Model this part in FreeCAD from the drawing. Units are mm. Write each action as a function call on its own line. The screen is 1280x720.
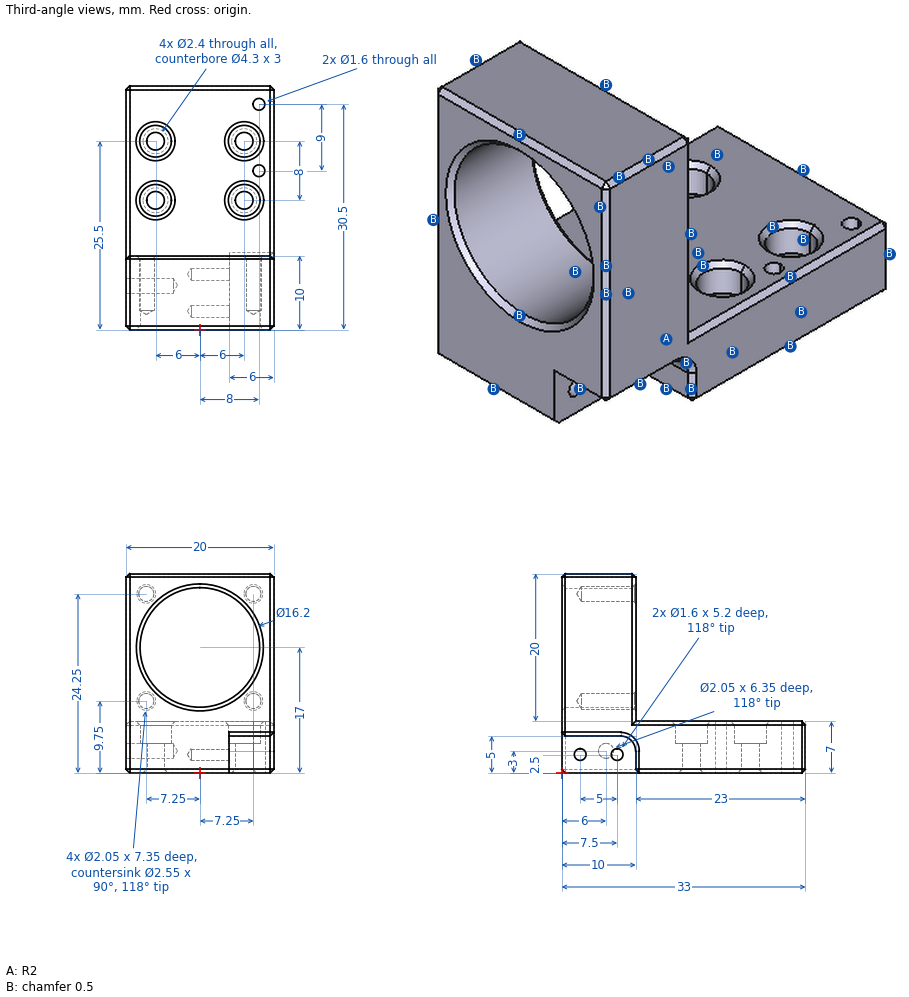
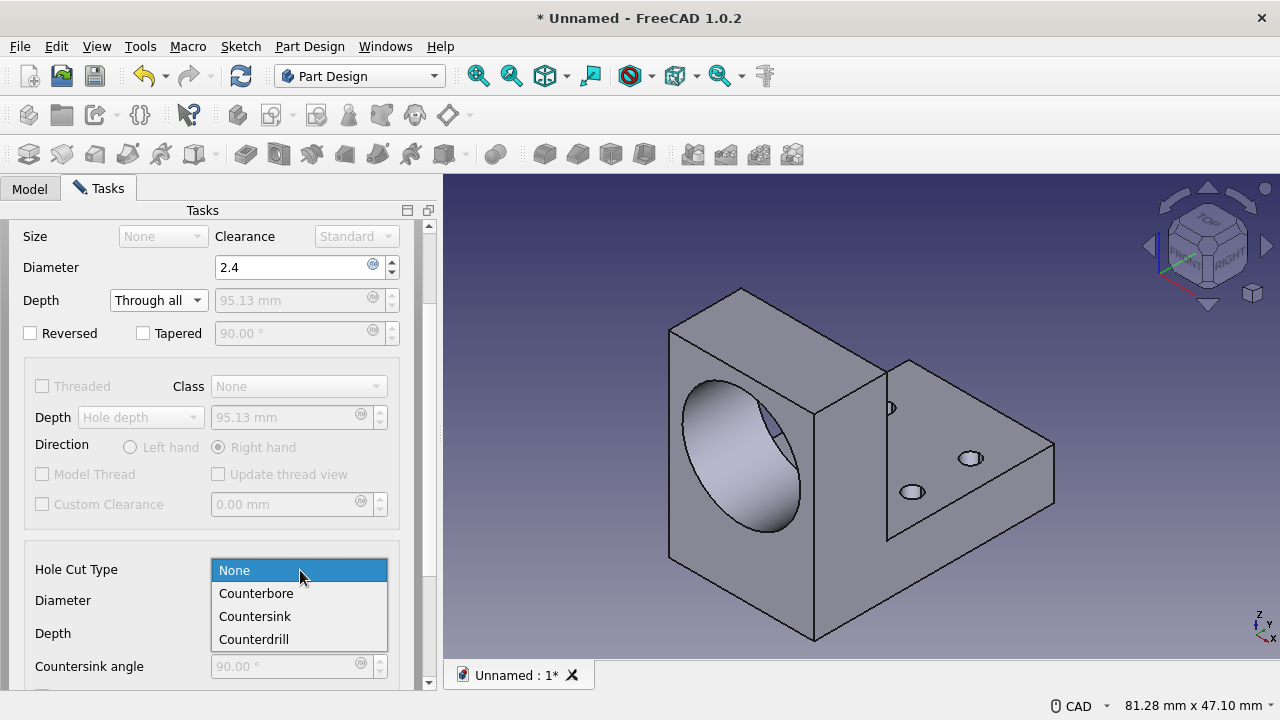
click(298, 594)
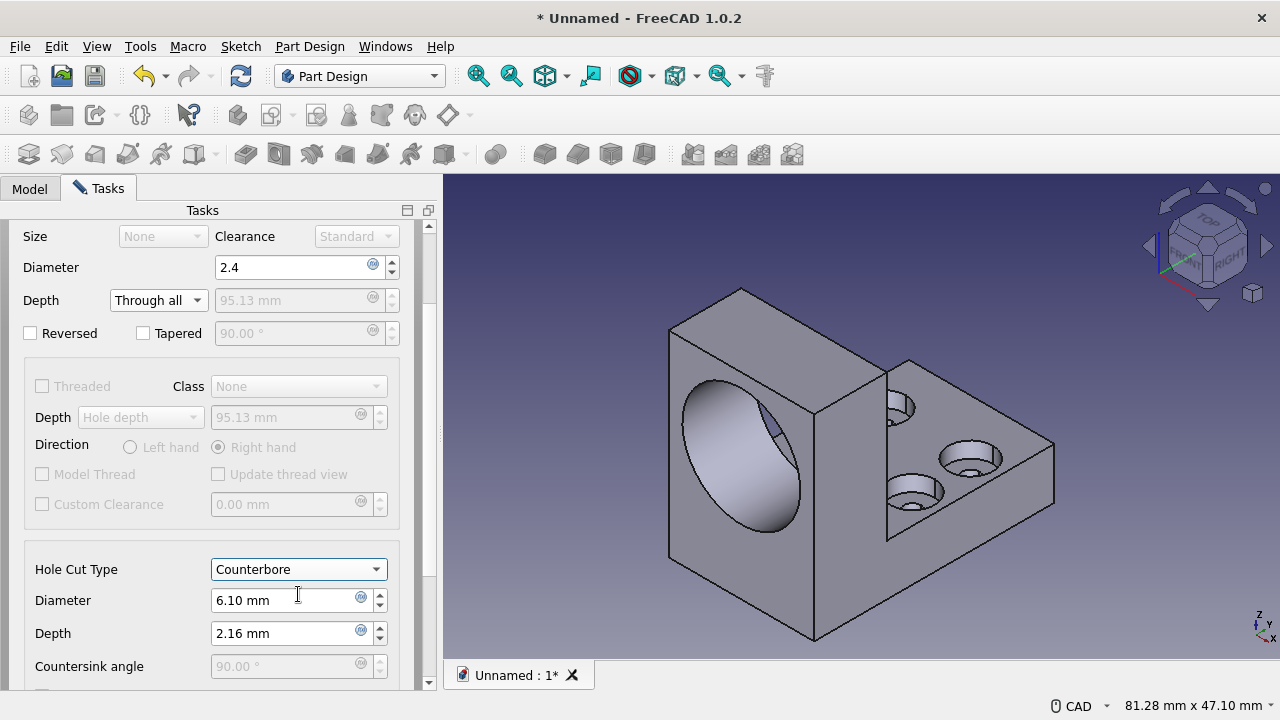
triple_click(292, 600)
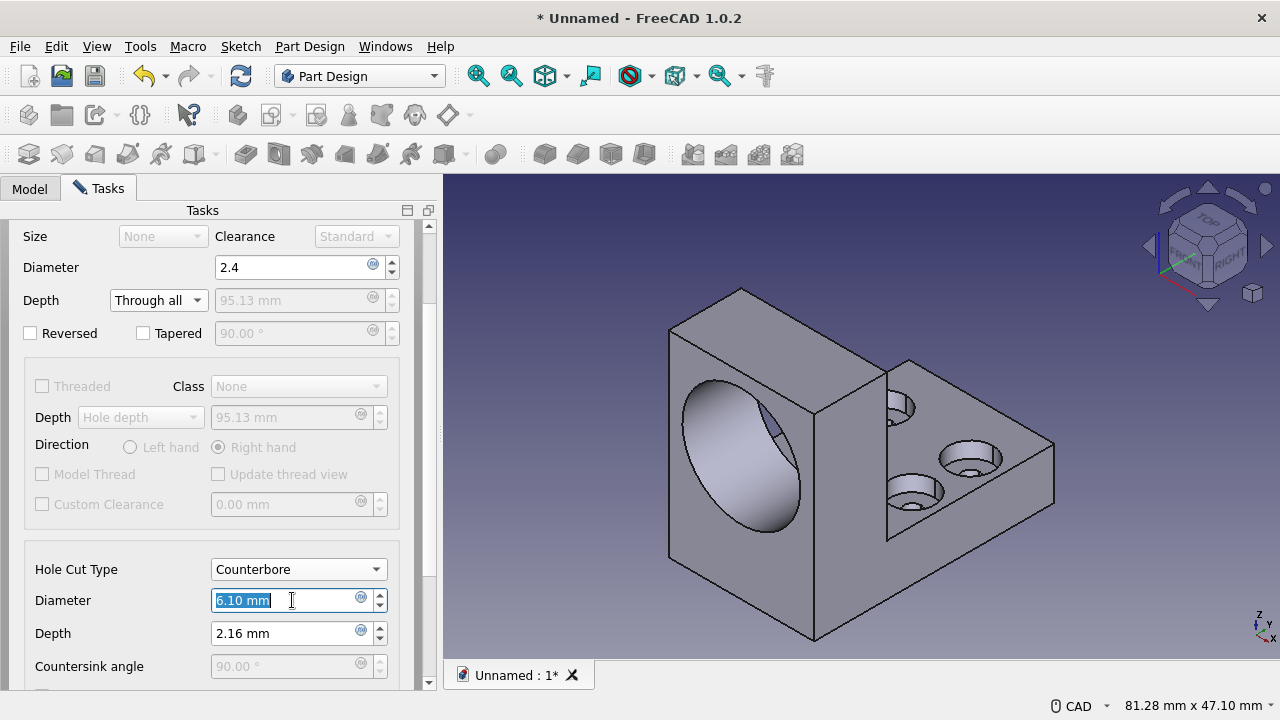
text(4.3)
key(Tab)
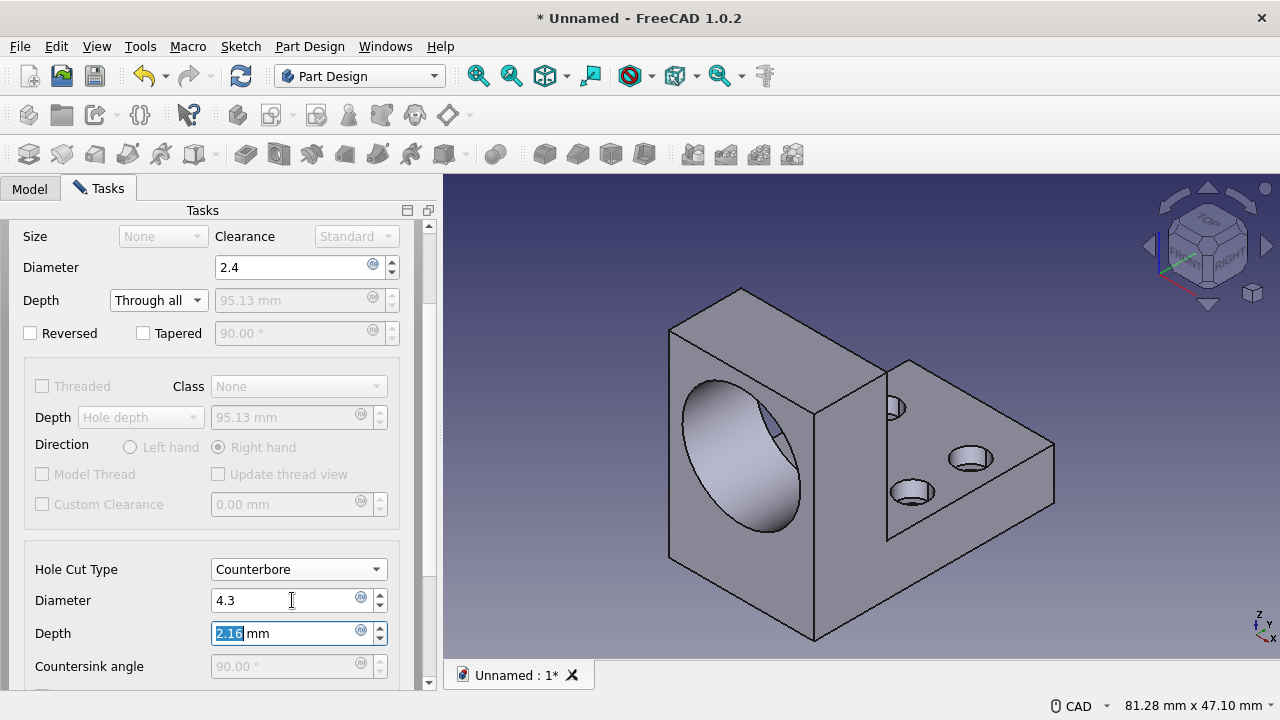
text(3)
key(Tab)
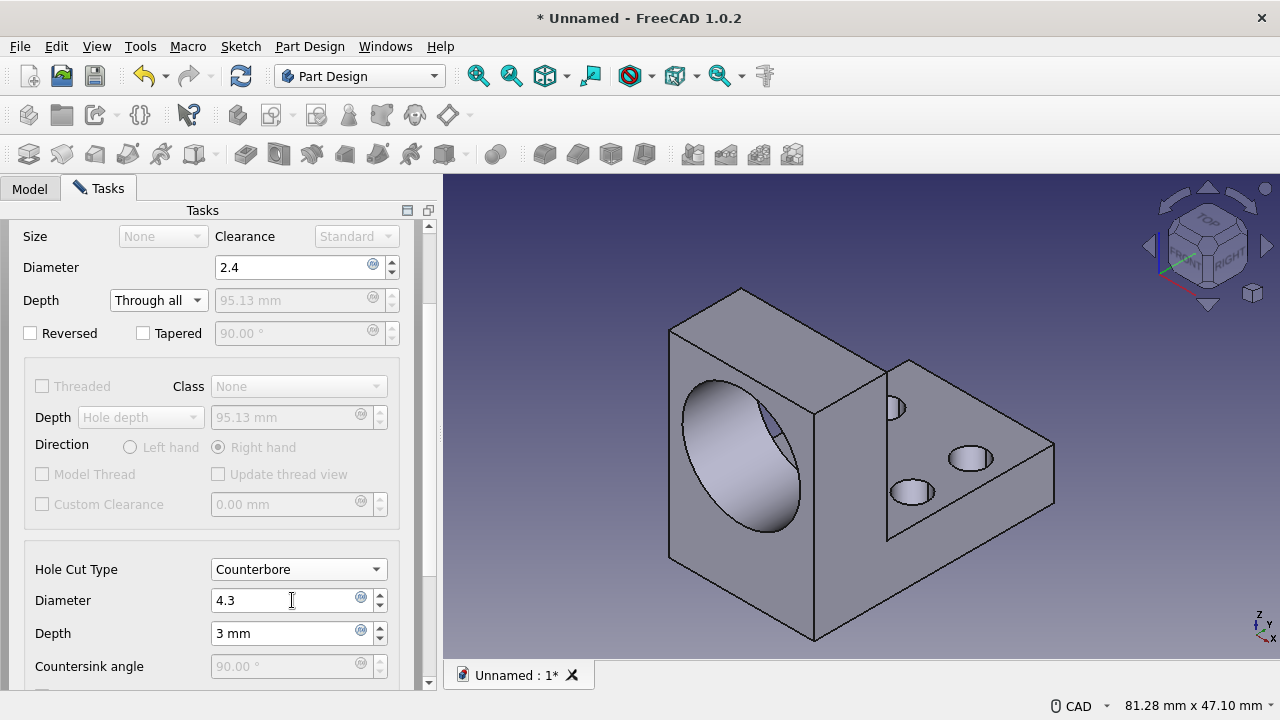
scroll(429, 455, up, 3)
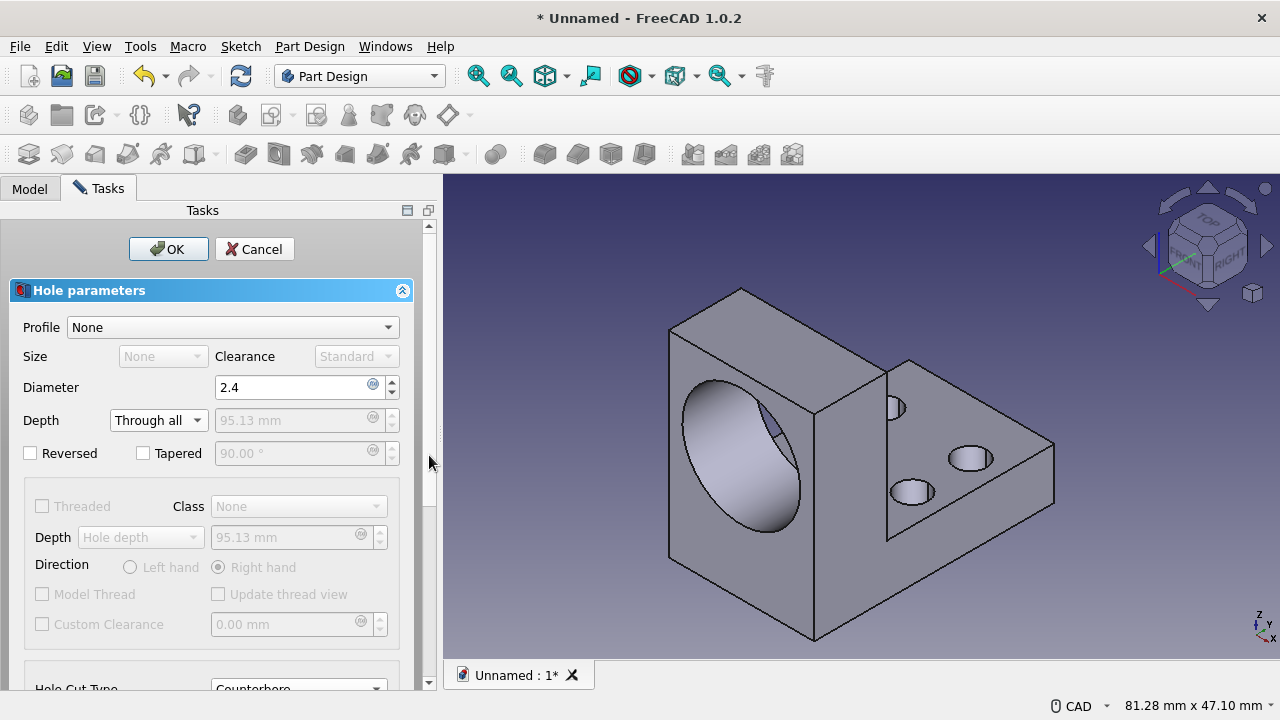
click(169, 249)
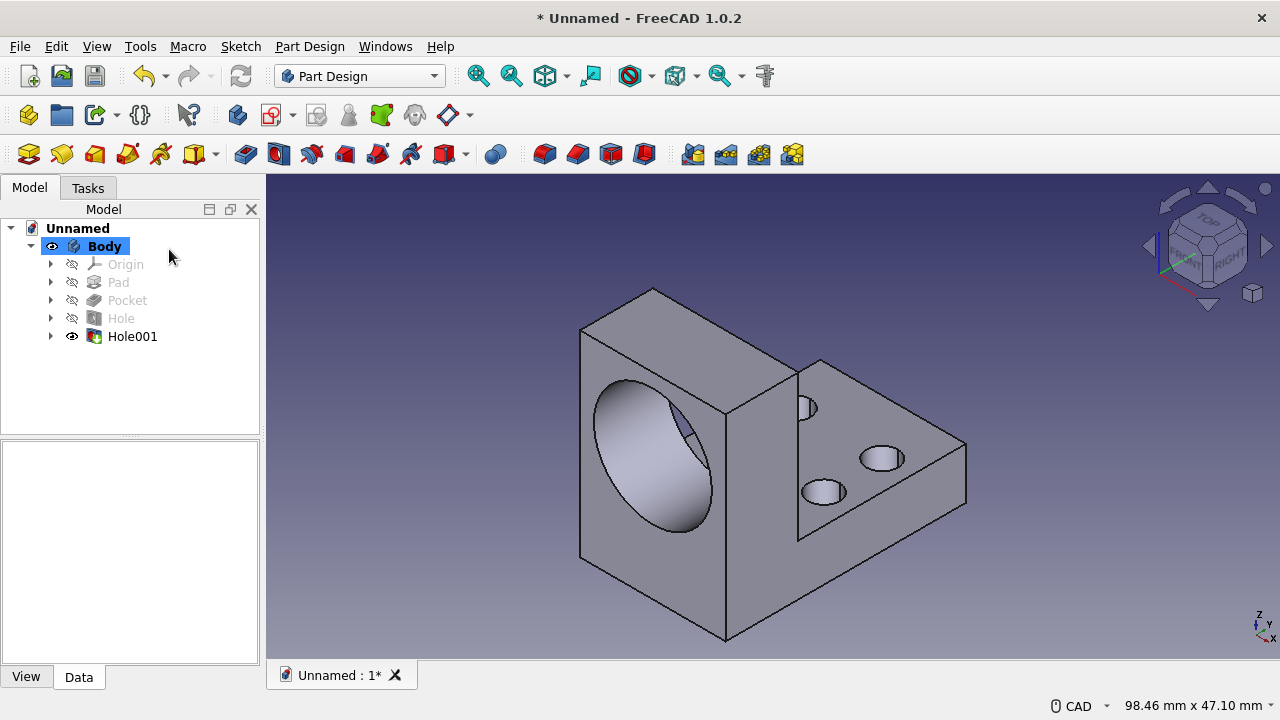
click(777, 562)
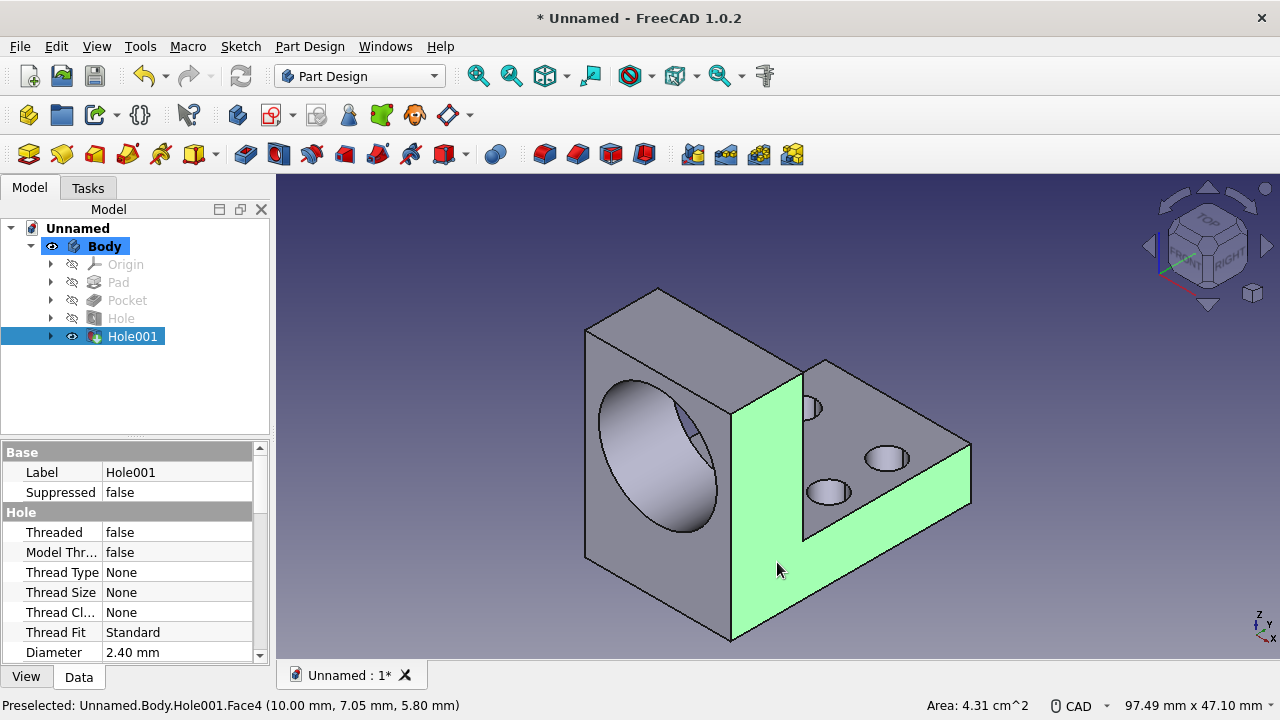
click(270, 116)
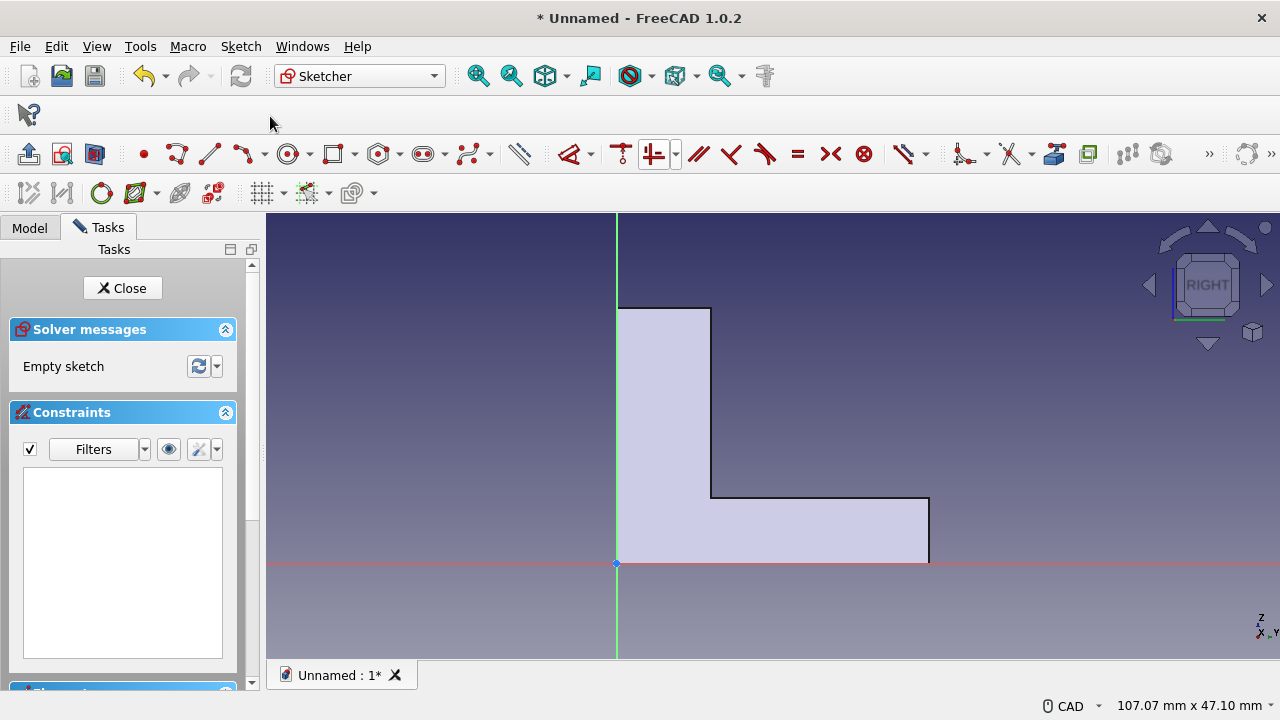
scroll(656, 561, up, 9)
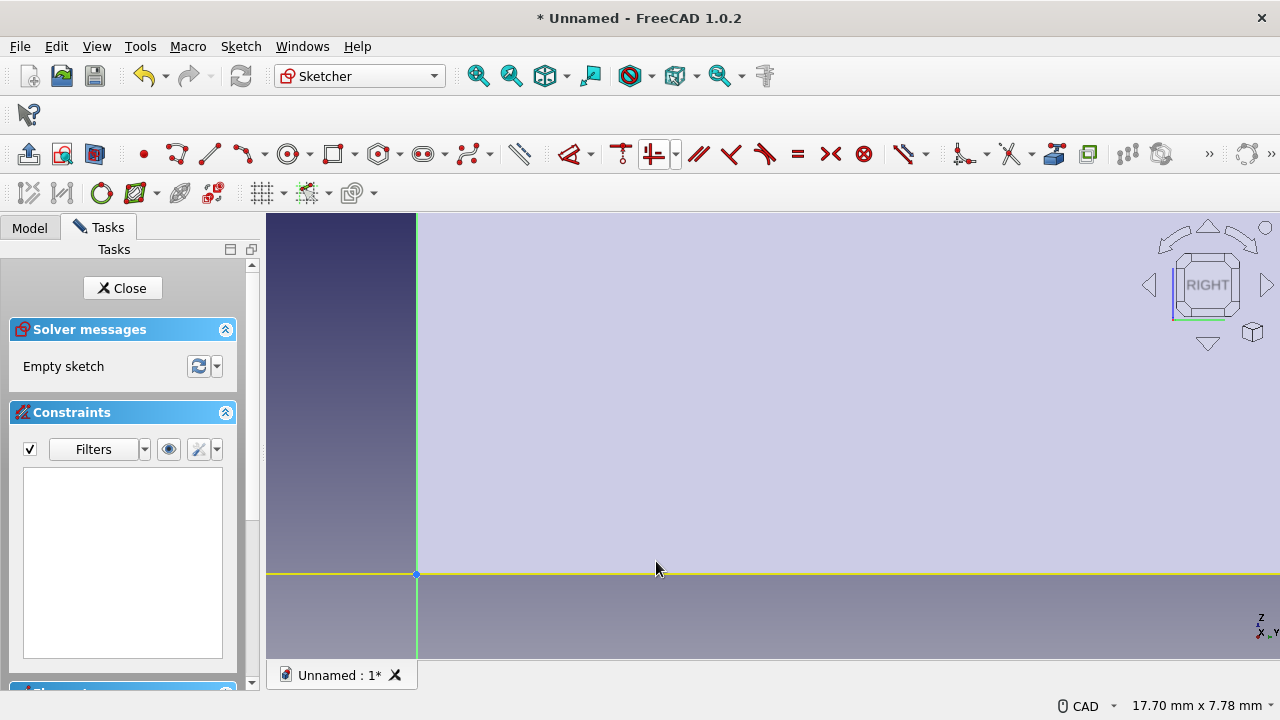
click(332, 154)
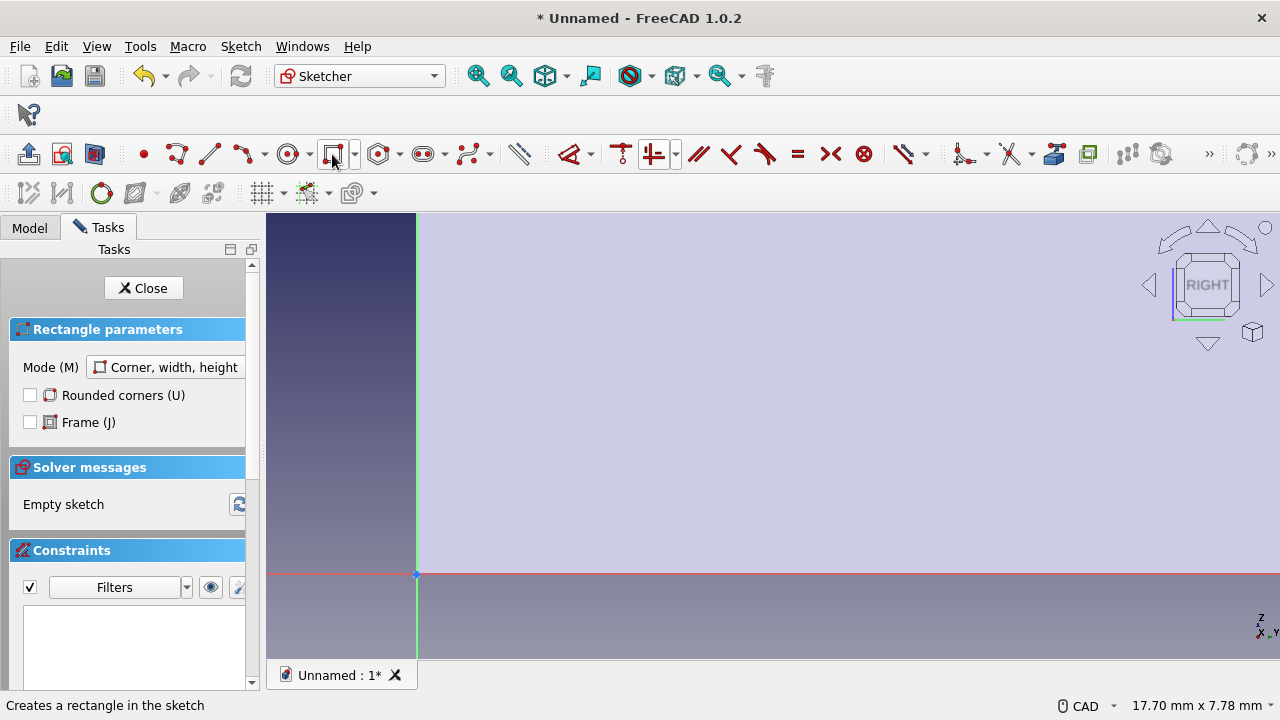
click(417, 574)
move(989, 288)